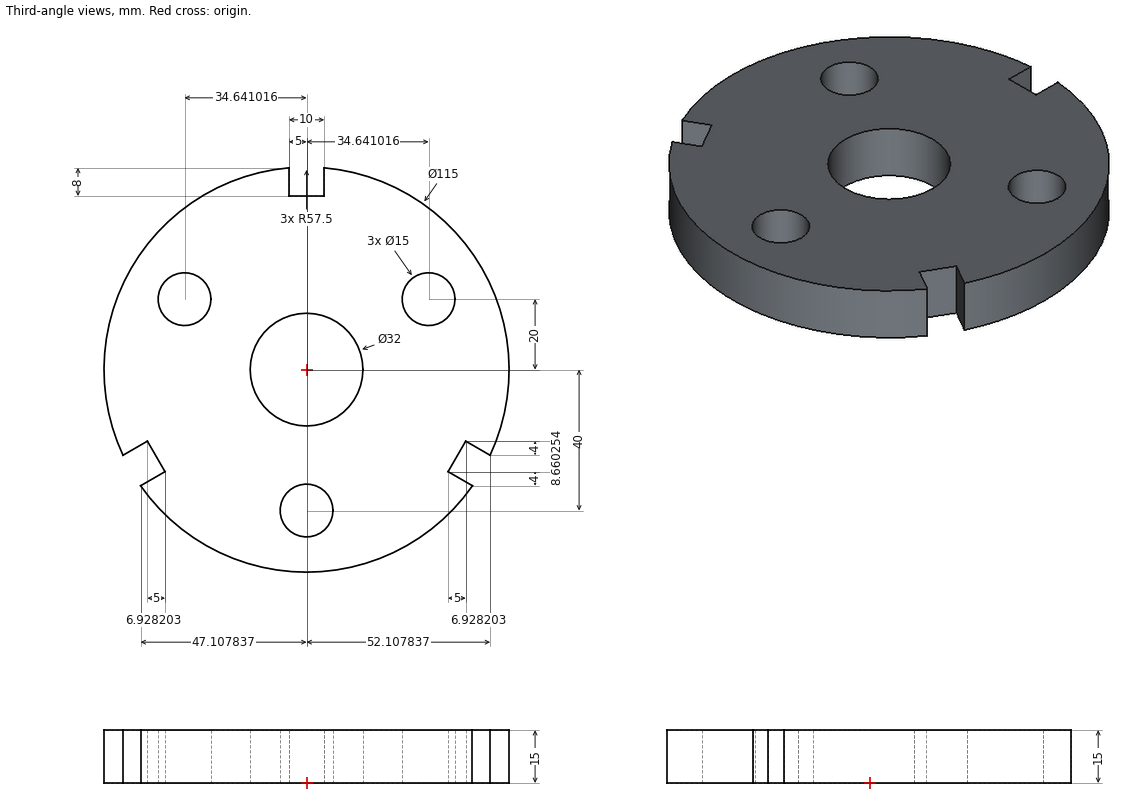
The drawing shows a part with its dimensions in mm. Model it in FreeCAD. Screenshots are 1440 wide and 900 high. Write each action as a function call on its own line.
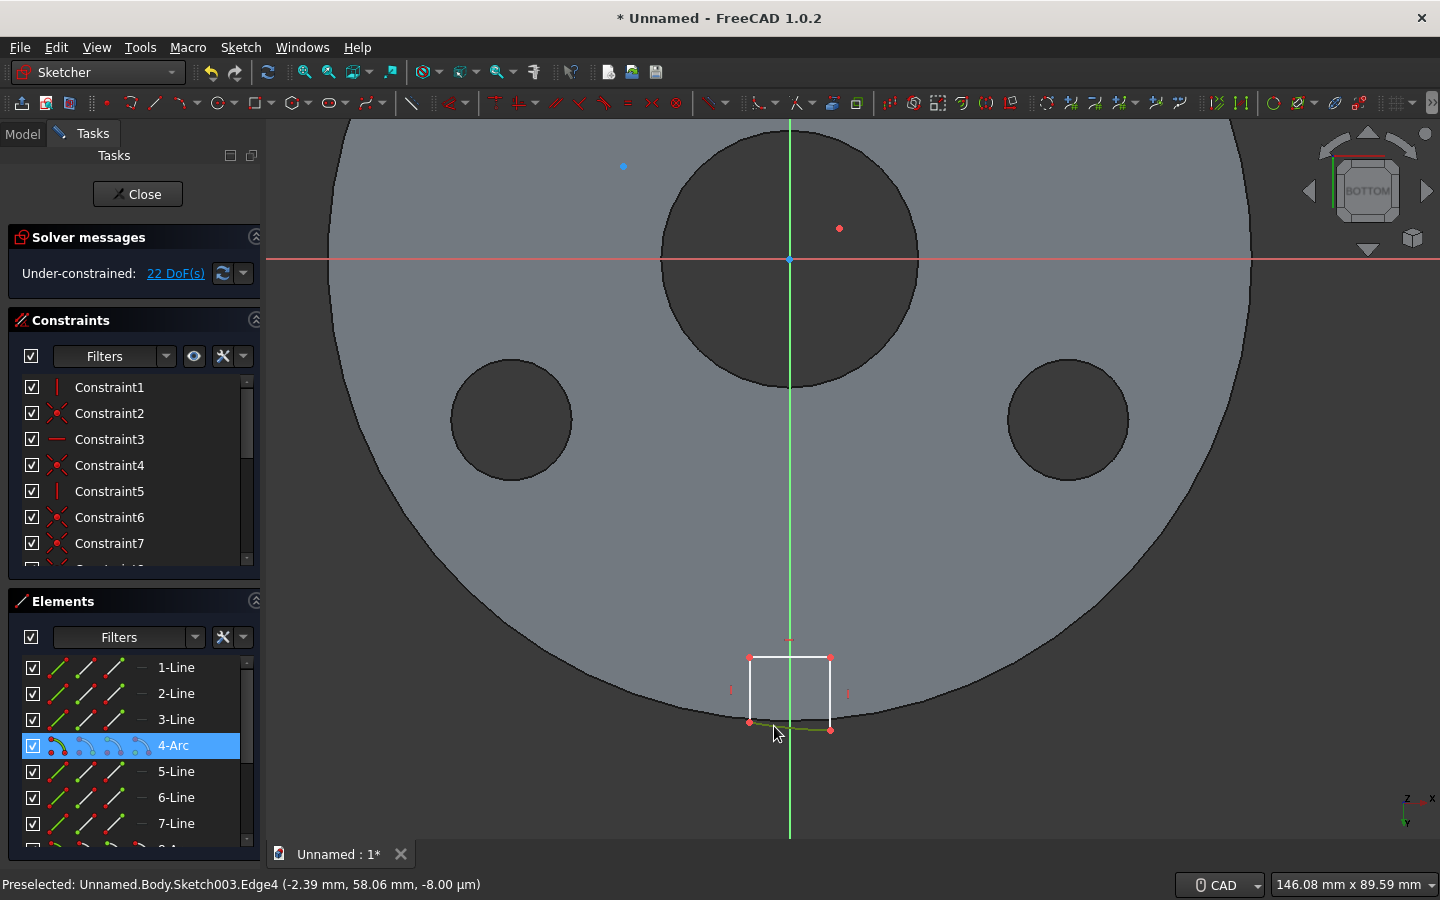
scroll(774, 726, down, 2)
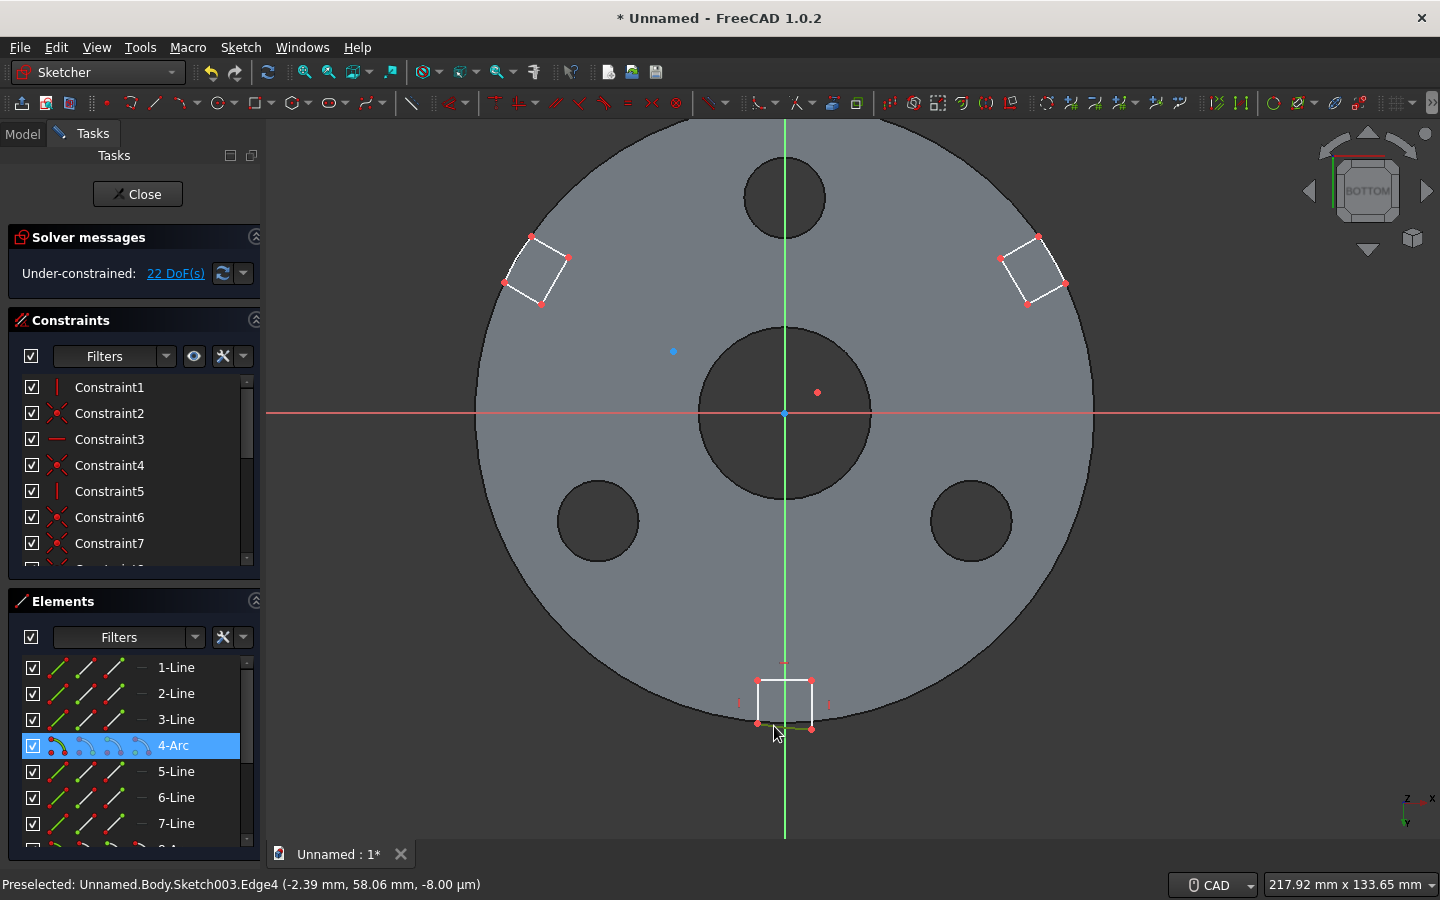
click(522, 250)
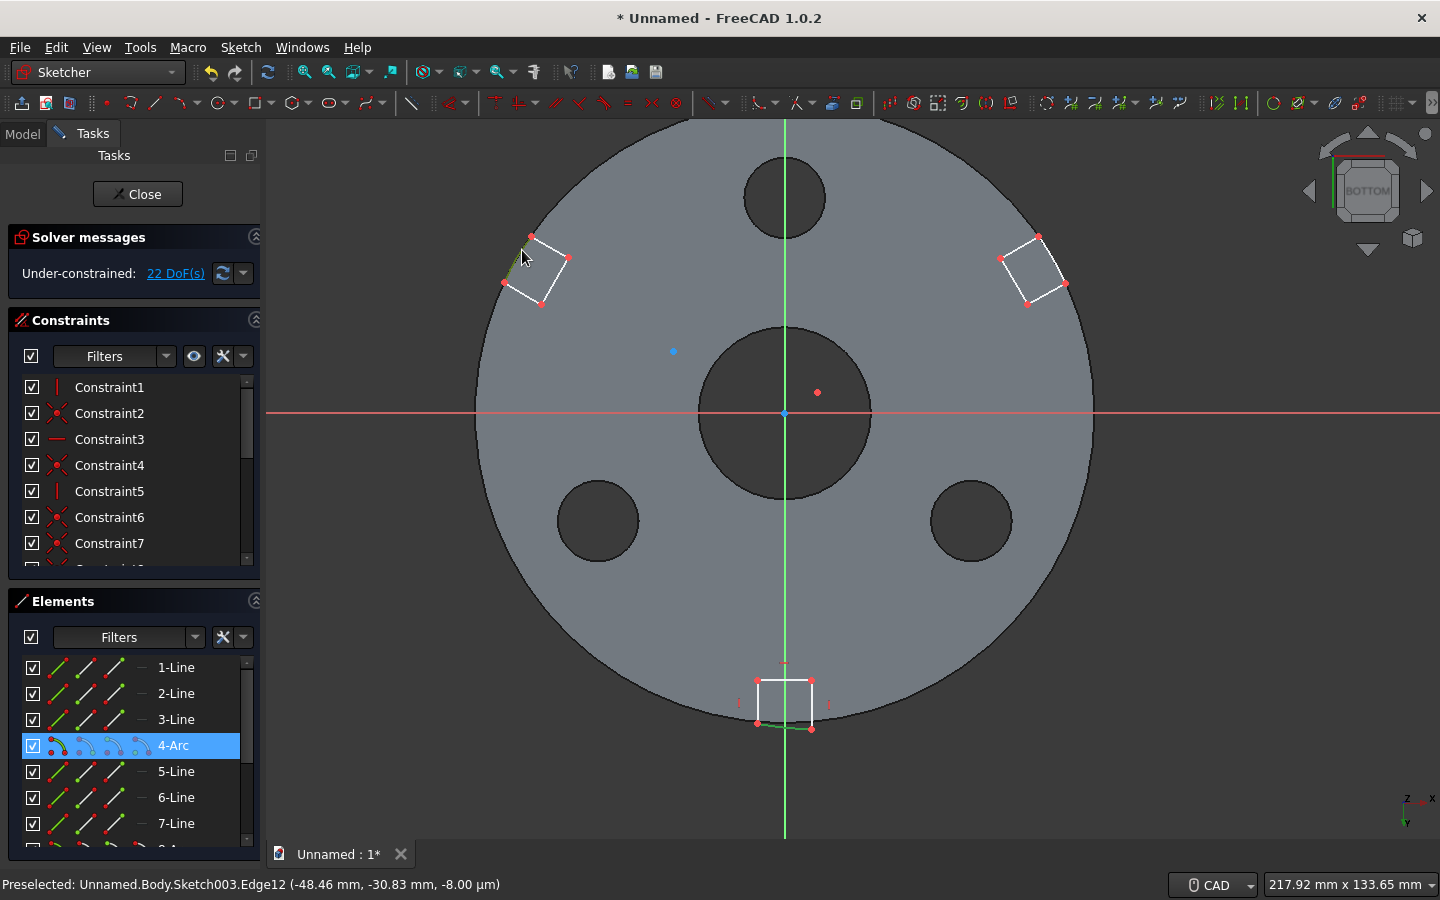
click(496, 104)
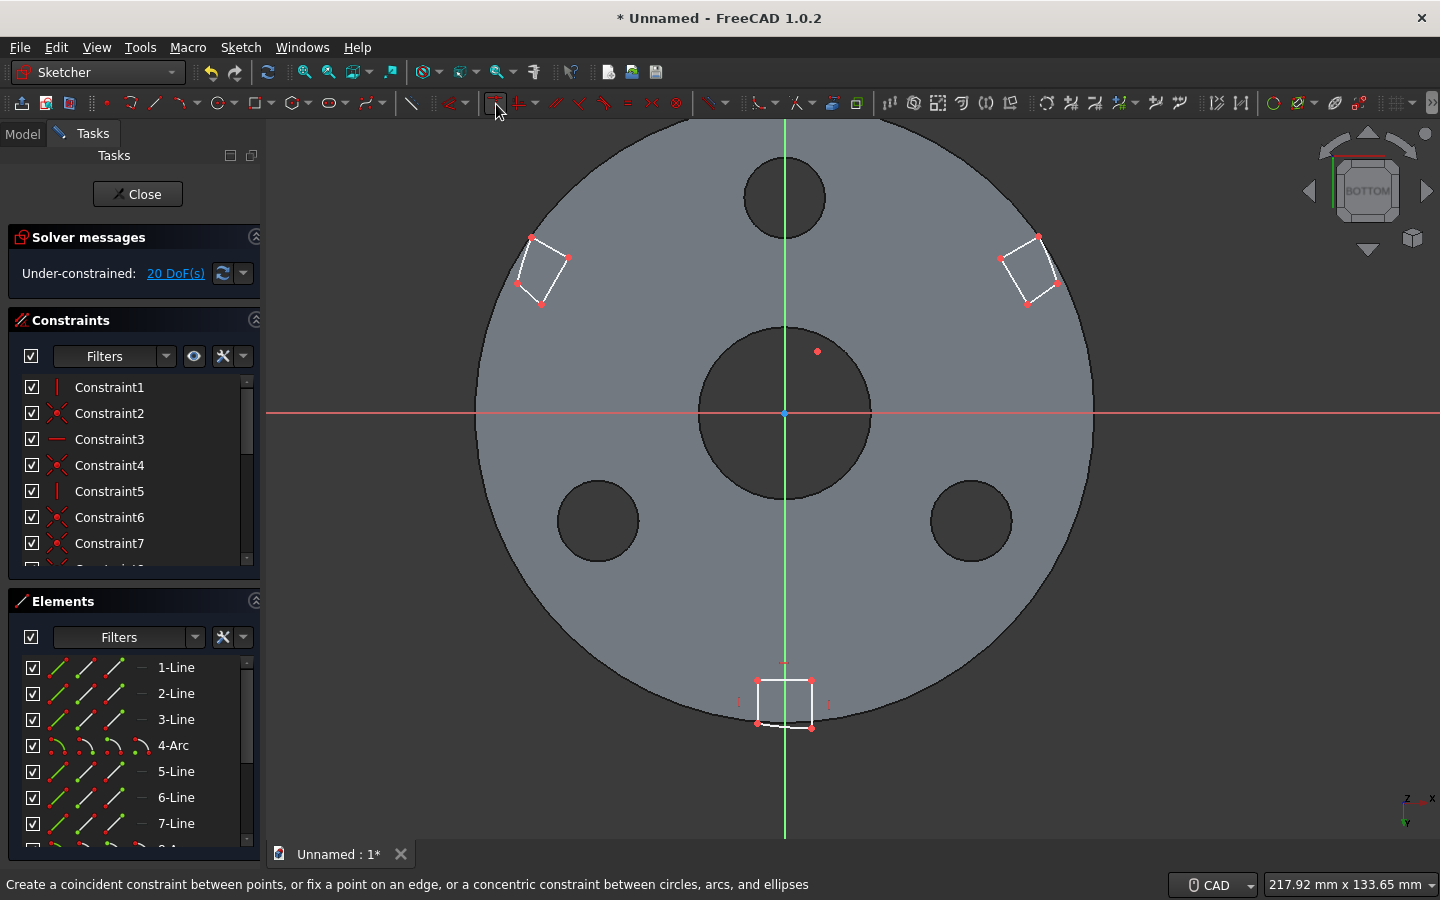
drag(775, 341, 827, 423)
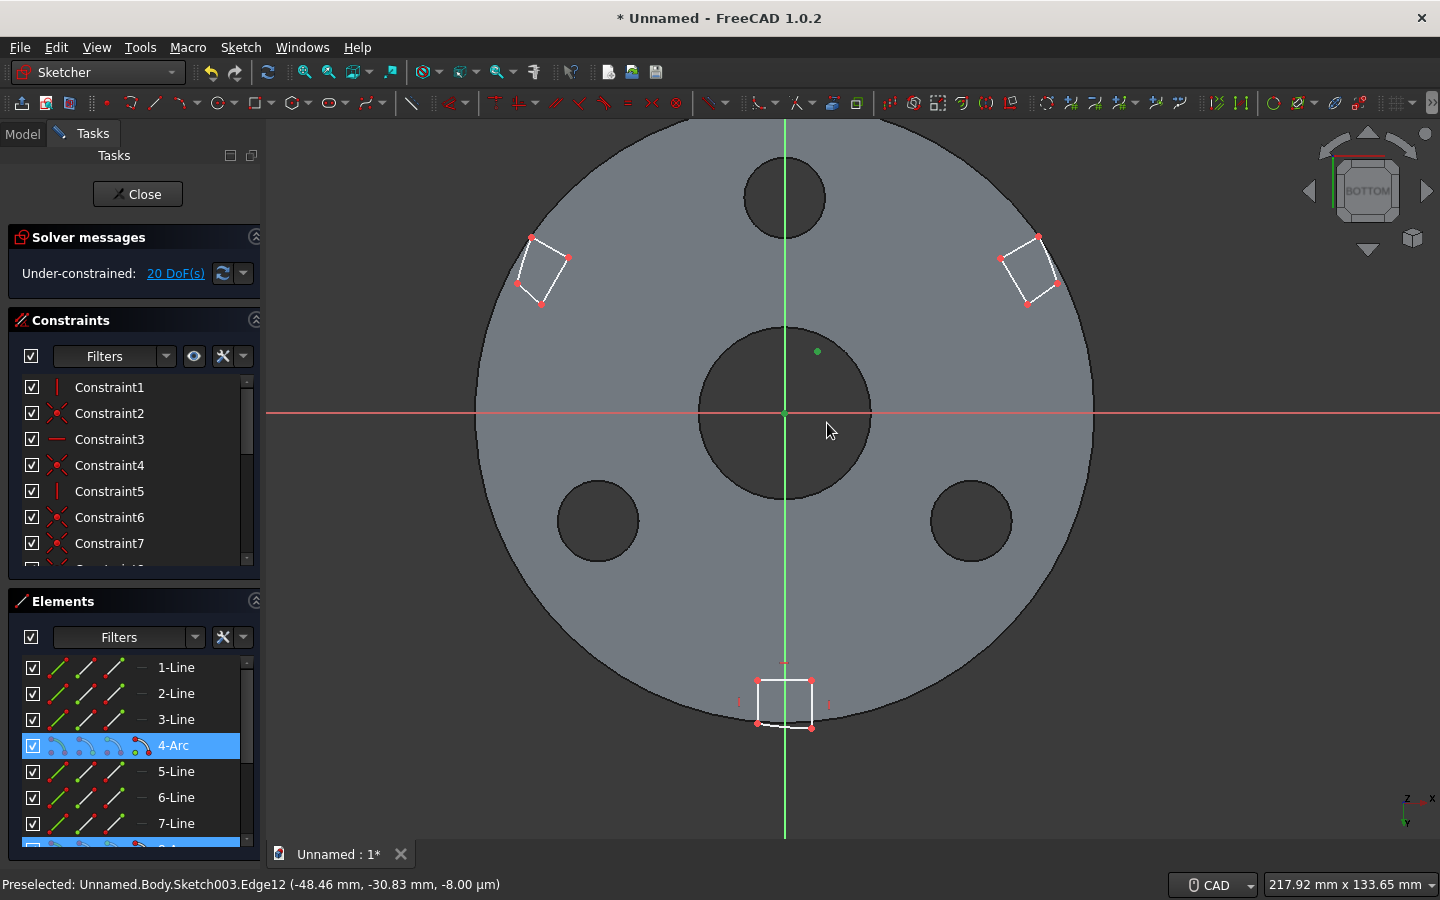
key(c)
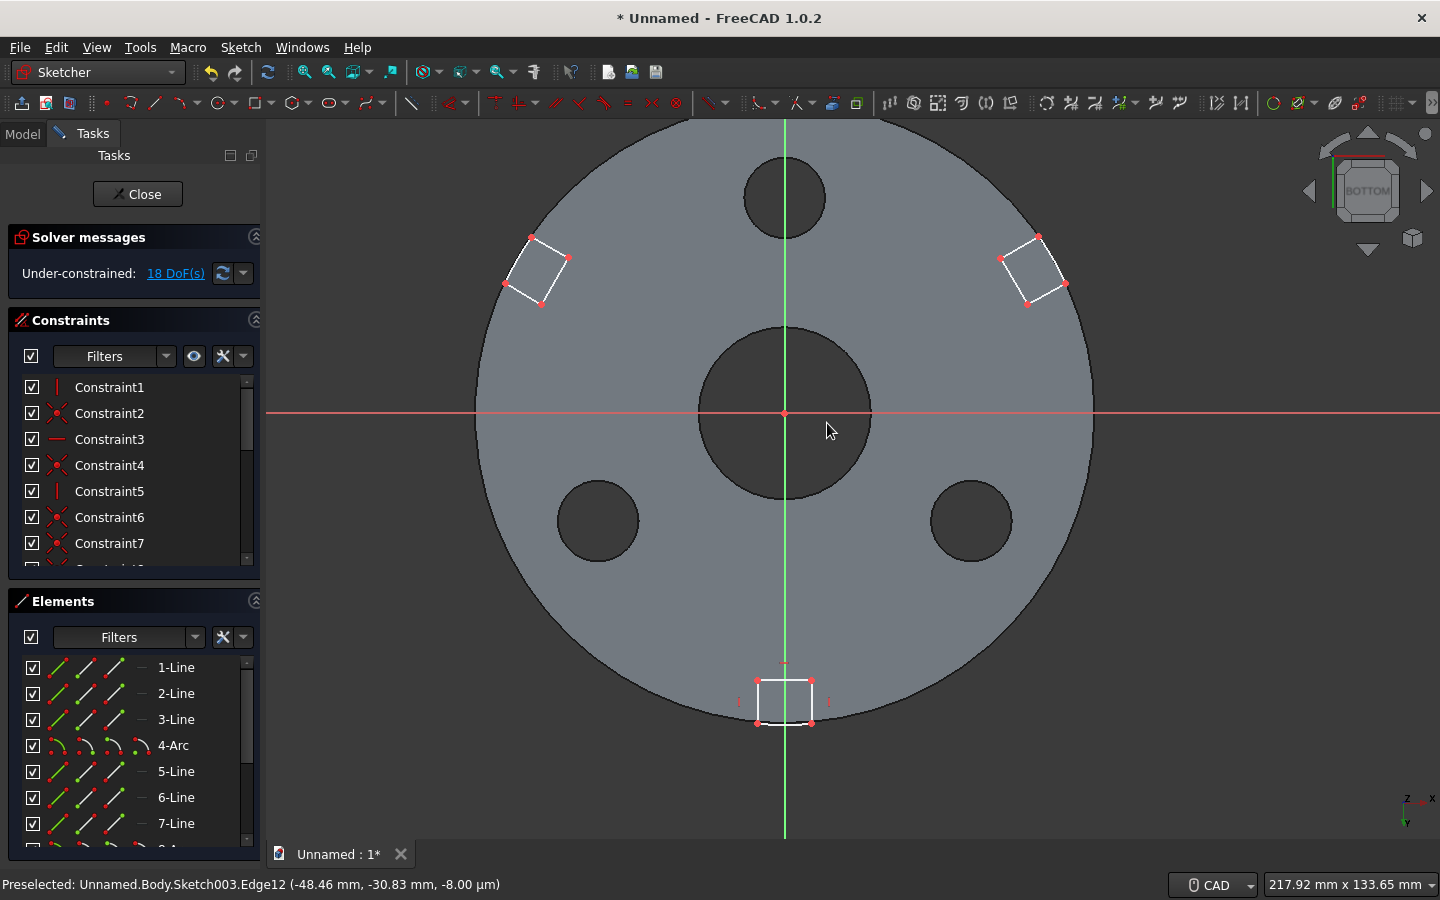
click(1059, 269)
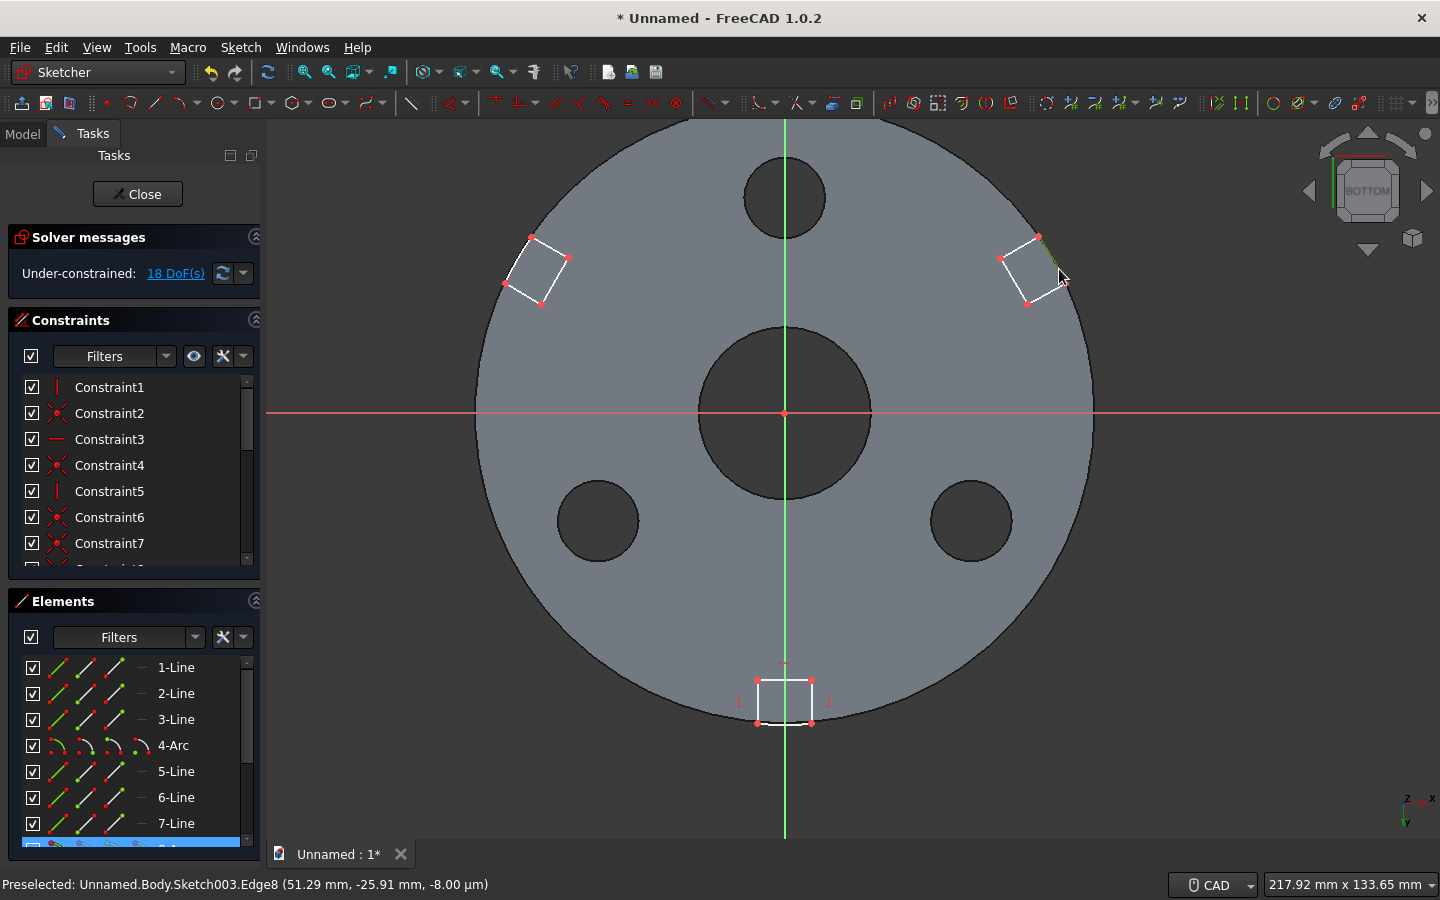
click(523, 250)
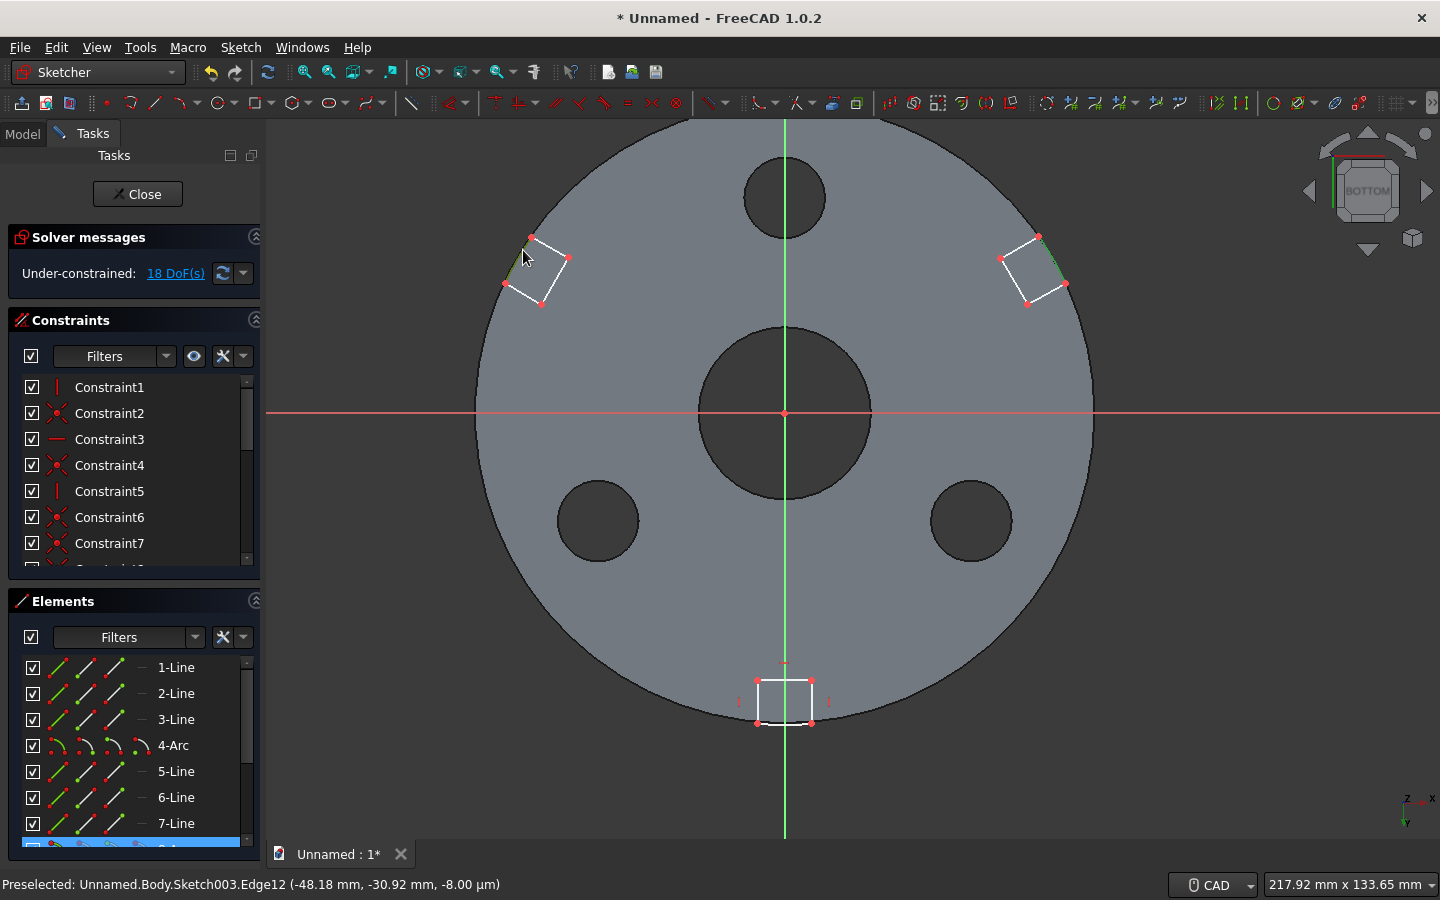
click(628, 104)